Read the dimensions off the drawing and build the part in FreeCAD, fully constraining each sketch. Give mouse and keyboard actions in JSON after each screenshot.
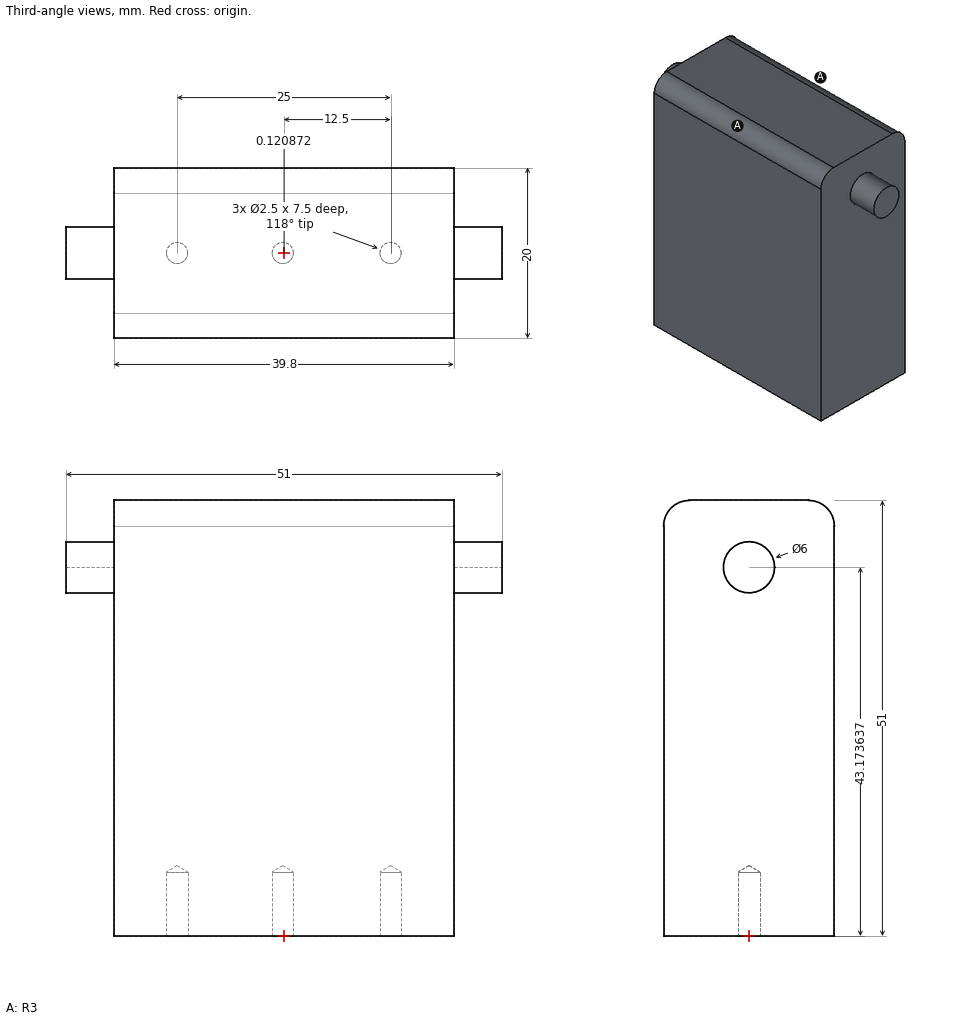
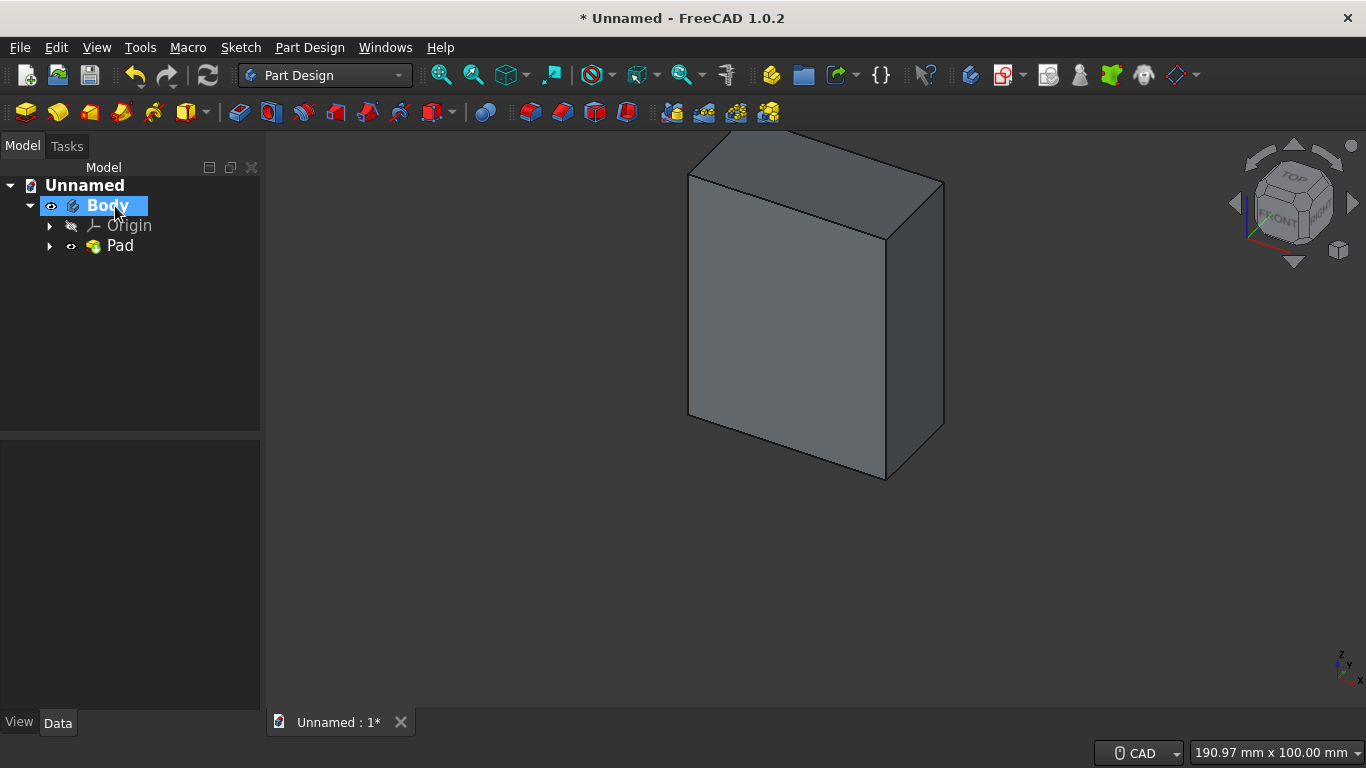
{"action": "key", "text": "v f"}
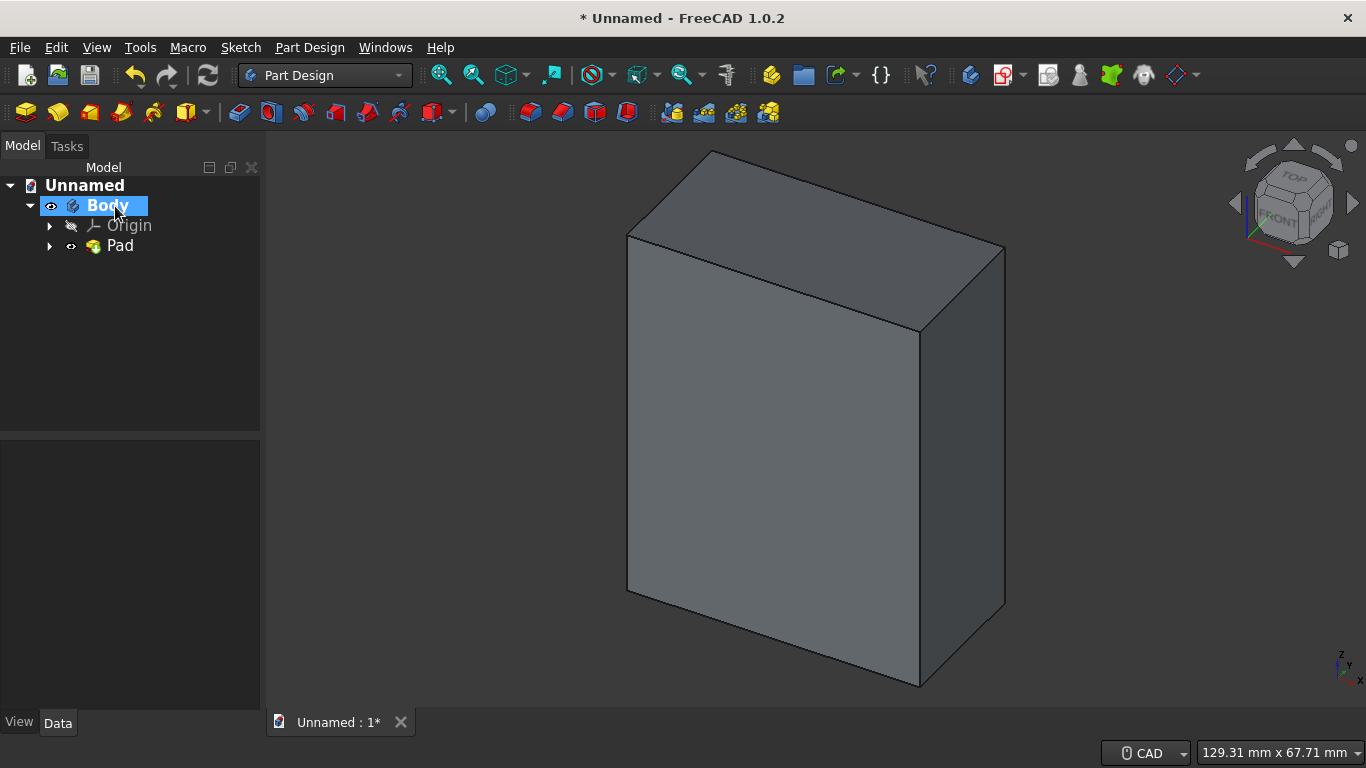
{"action": "left_click", "coordinate": [1004, 76]}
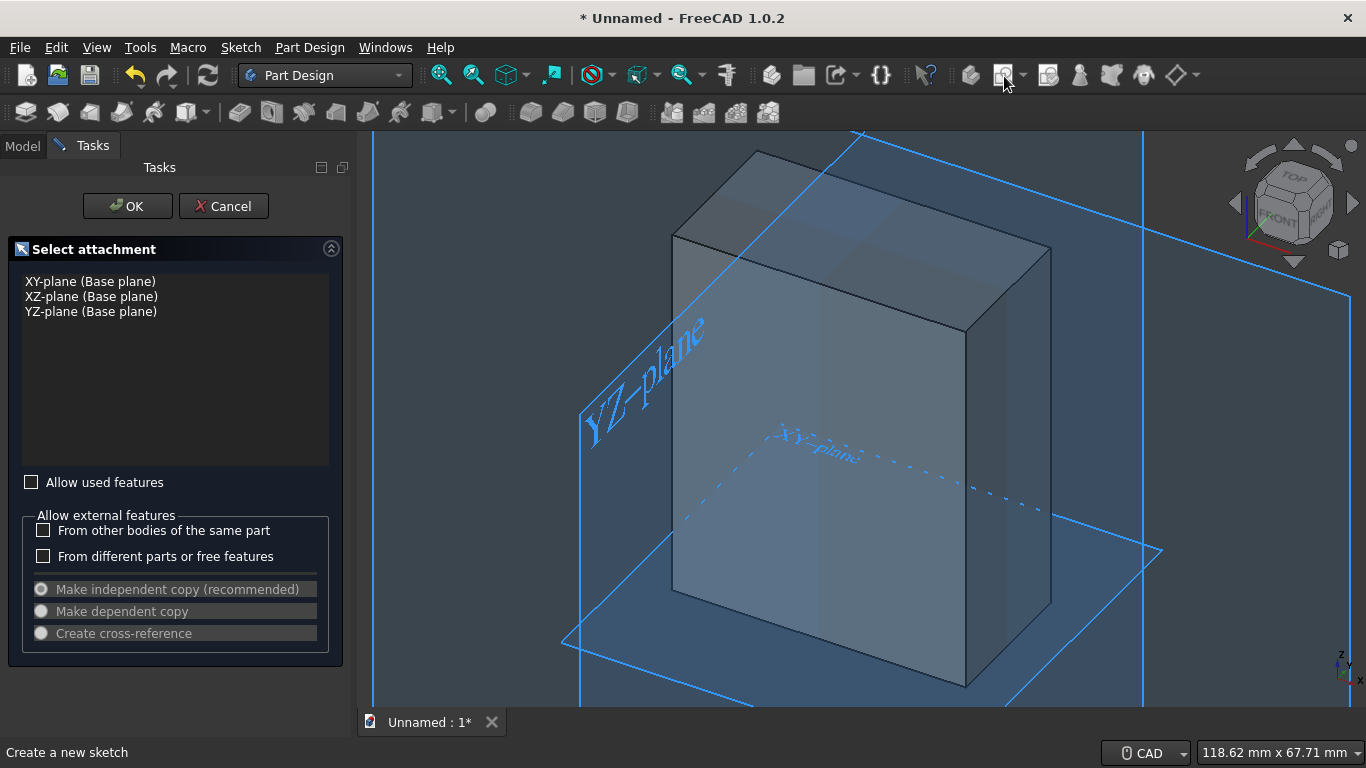
{"action": "left_click", "coordinate": [82, 312]}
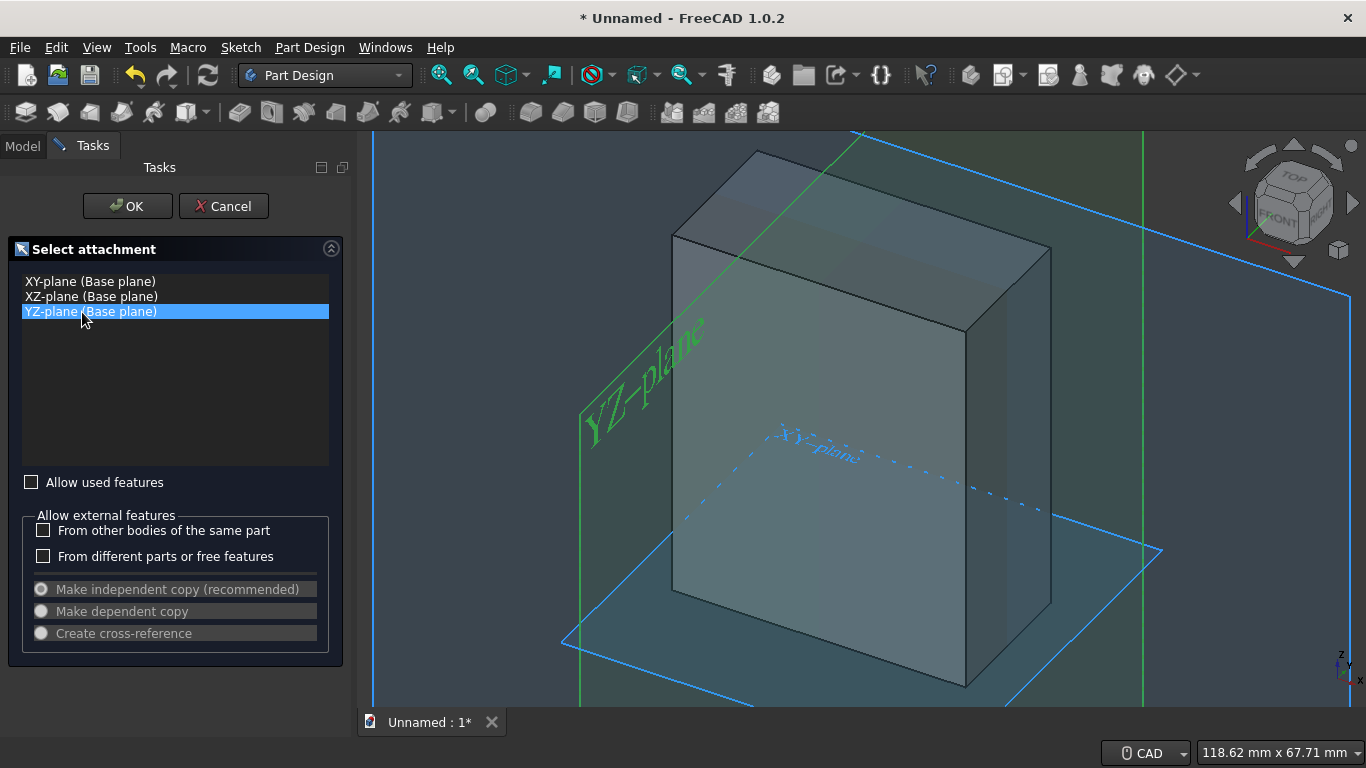
{"action": "left_click", "coordinate": [128, 206]}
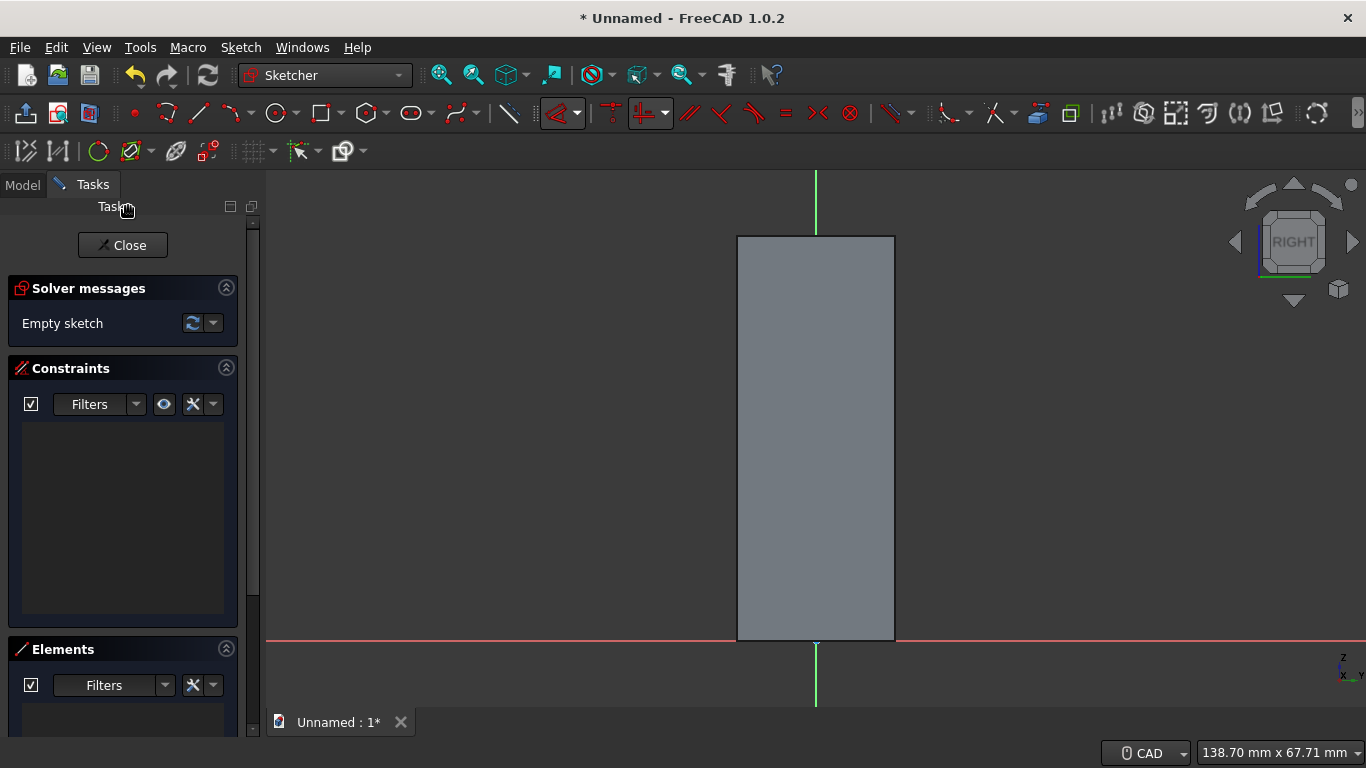
{"action": "key", "text": "q s"}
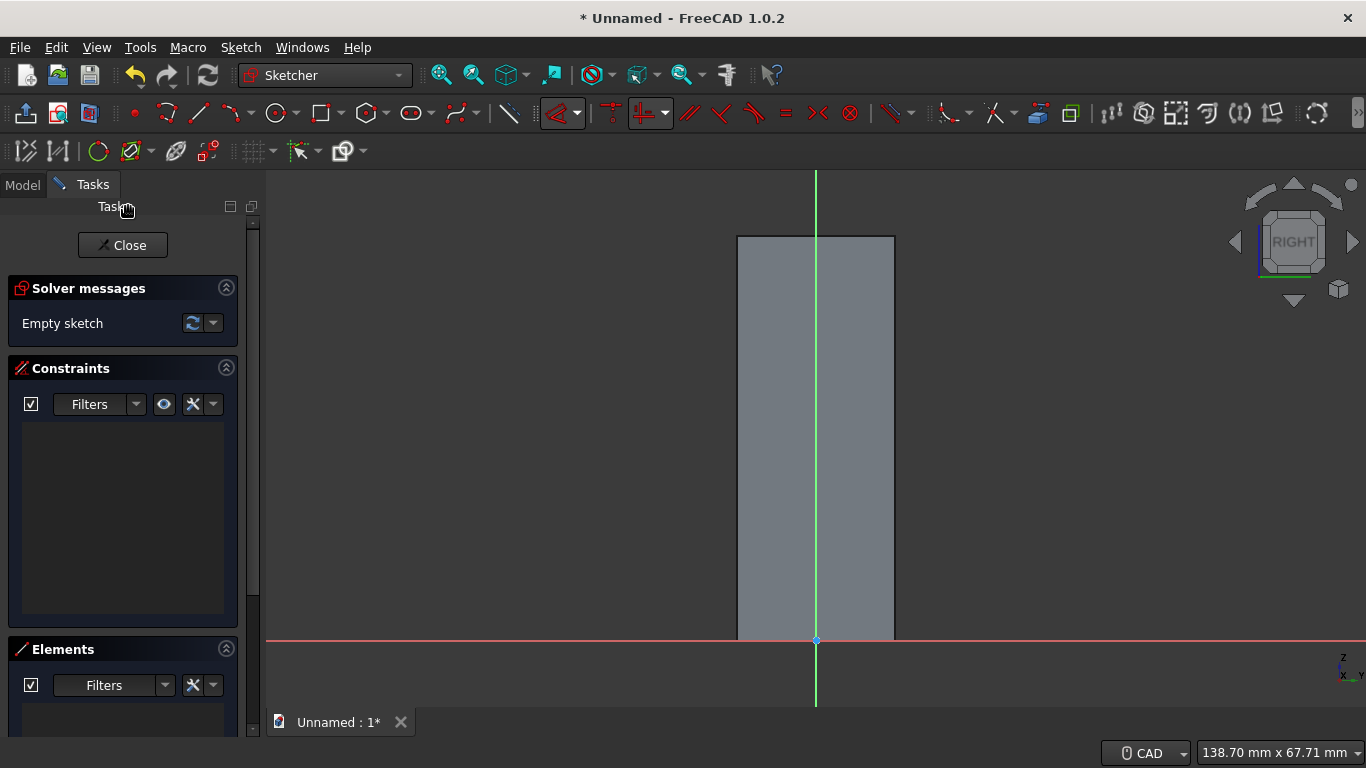
{"action": "scroll", "coordinate": [827, 276], "scroll_direction": "up", "scroll_amount": 10}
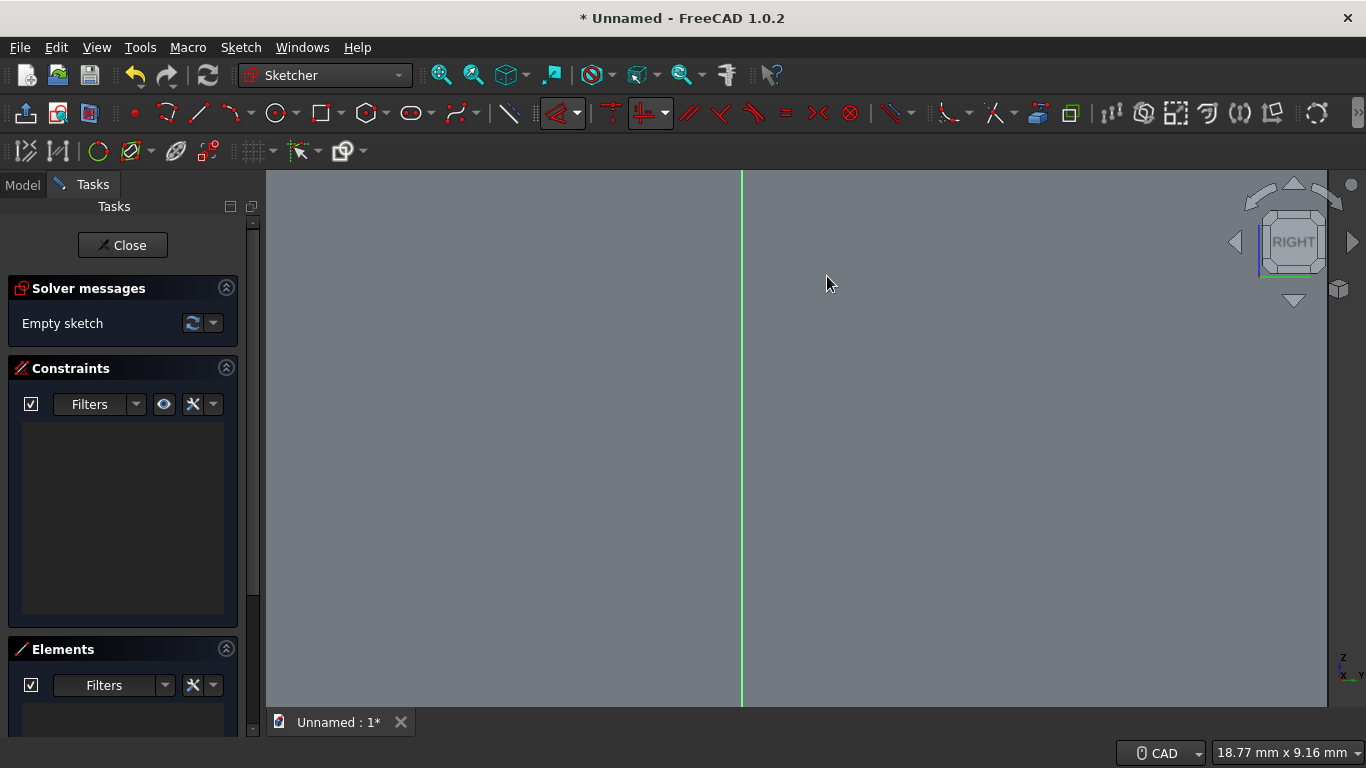
{"action": "left_click", "coordinate": [276, 114]}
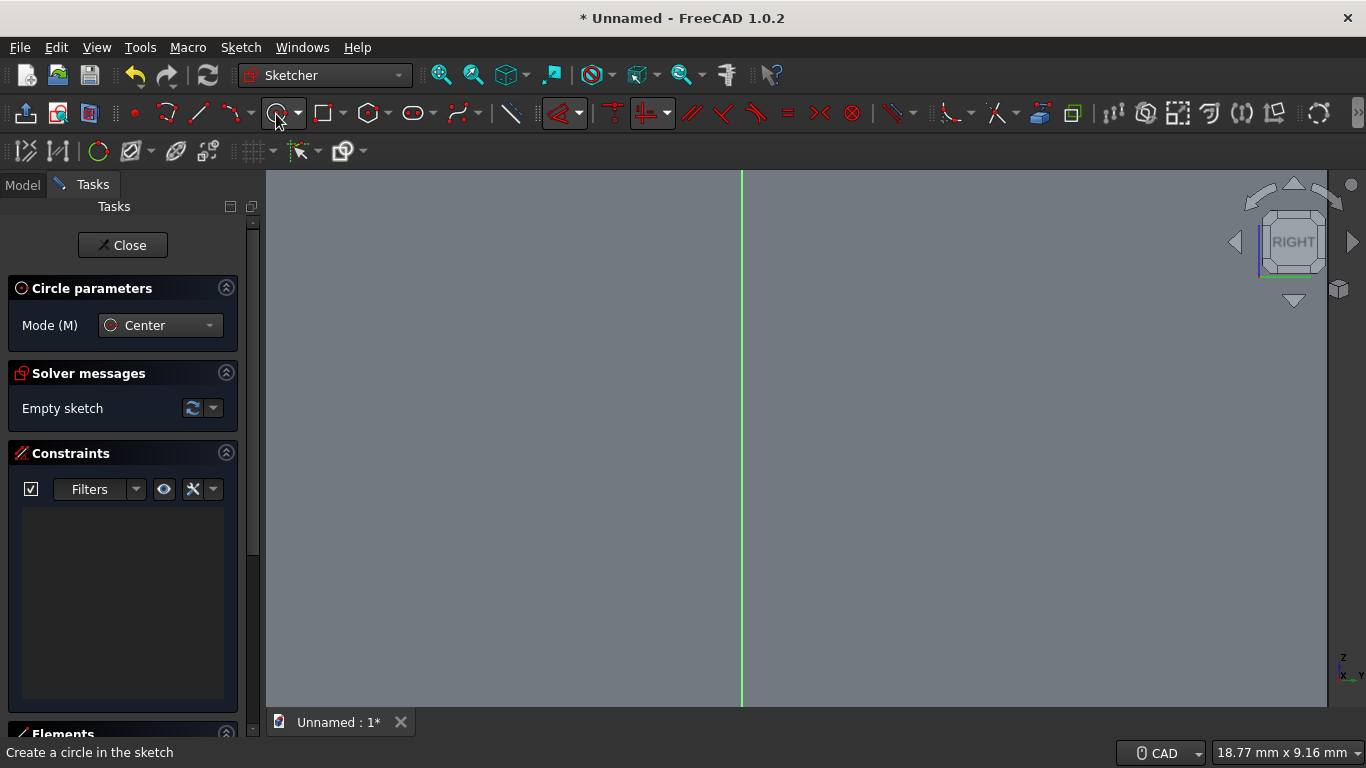
{"action": "left_click", "coordinate": [742, 440]}
{"action": "left_click", "coordinate": [867, 315]}
{"action": "key", "text": "Escape"}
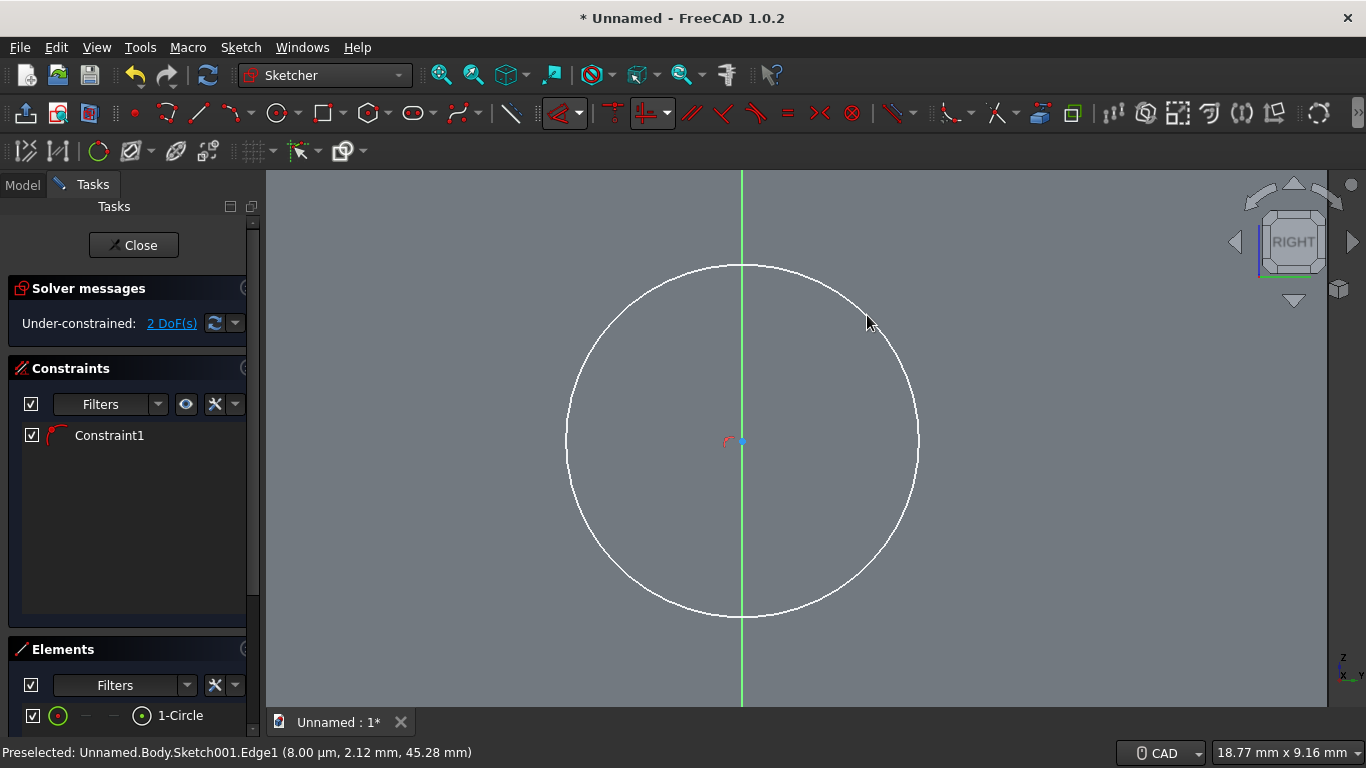
{"action": "left_click", "coordinate": [867, 316]}